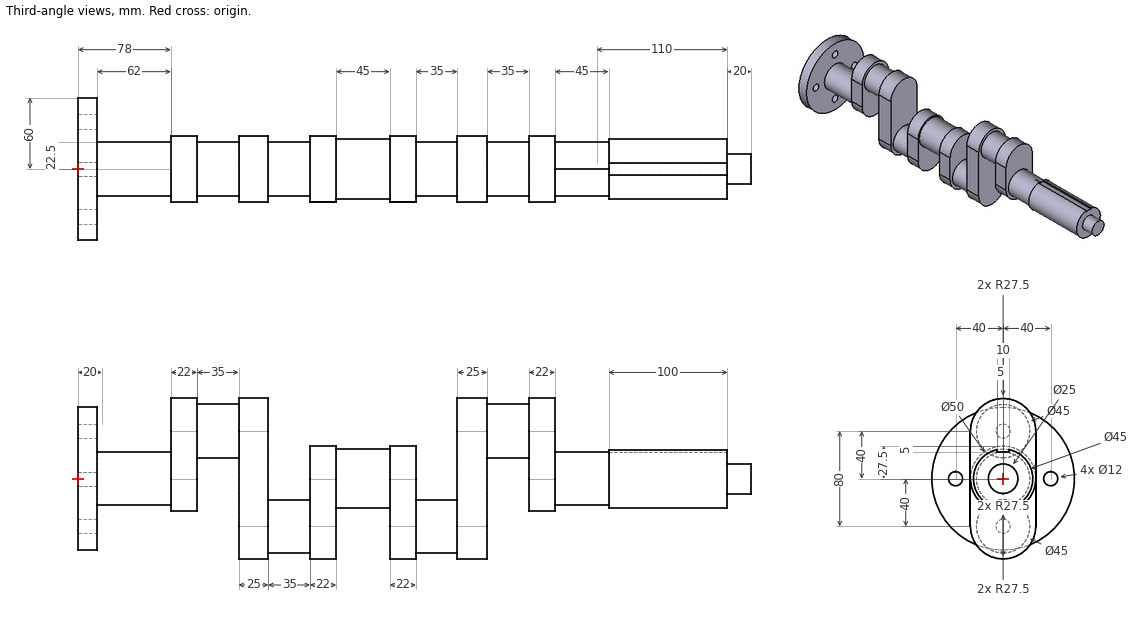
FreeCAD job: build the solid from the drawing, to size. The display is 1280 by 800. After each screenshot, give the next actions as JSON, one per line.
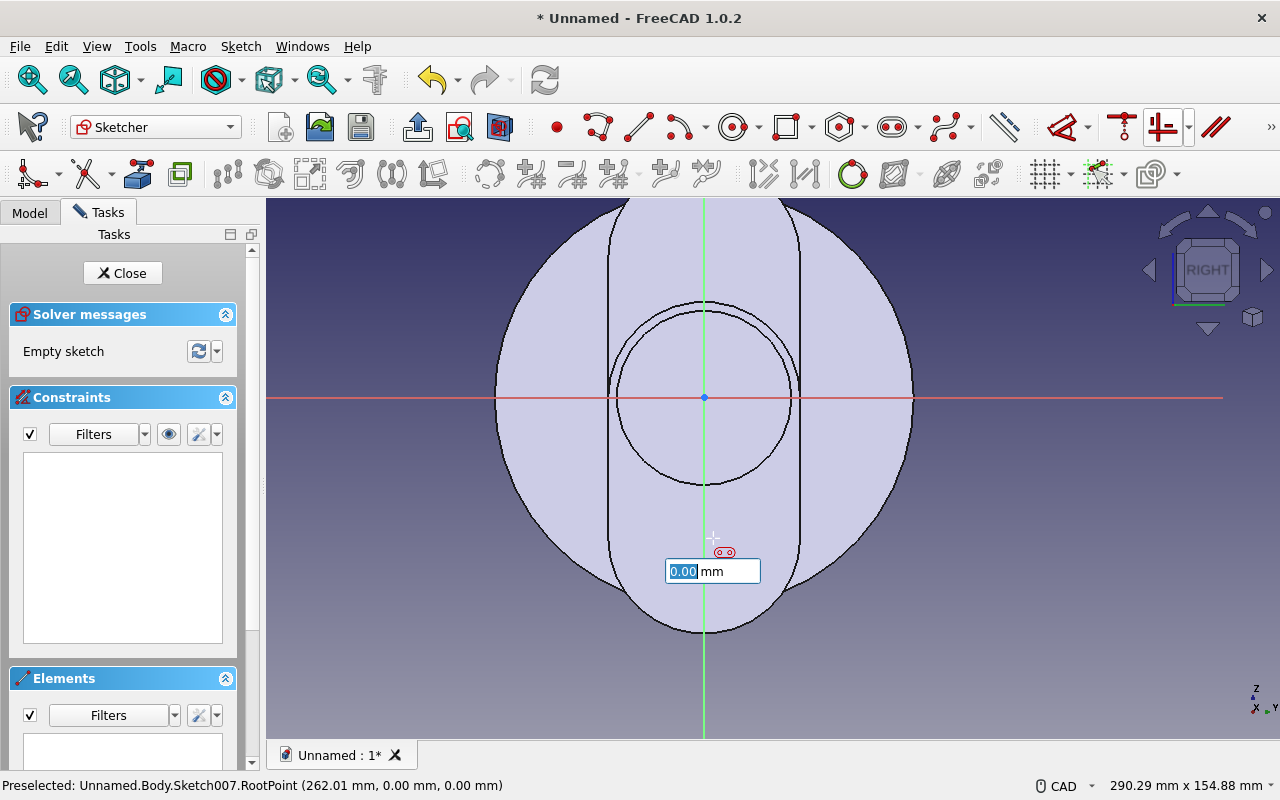
{"action": "left_click", "coordinate": [800, 468]}
{"action": "key", "text": "Escape"}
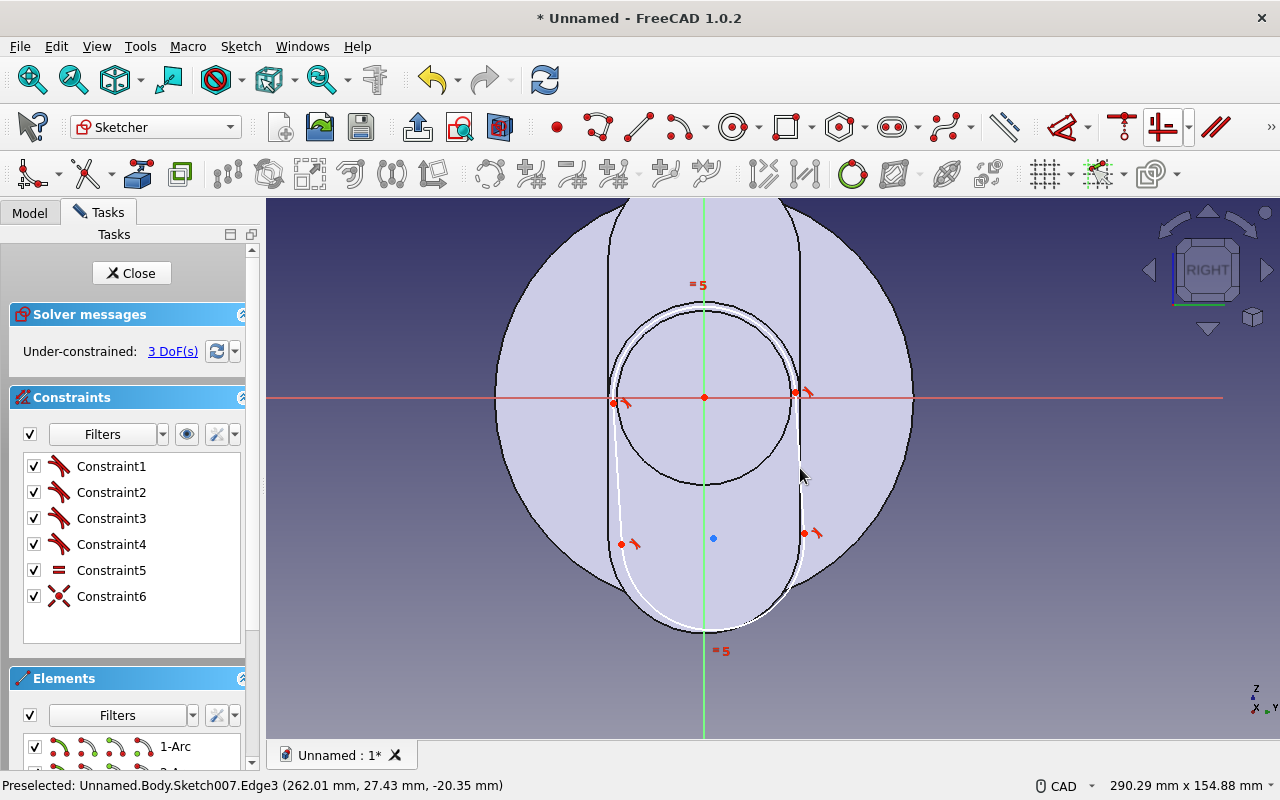
{"action": "left_click", "coordinate": [798, 435]}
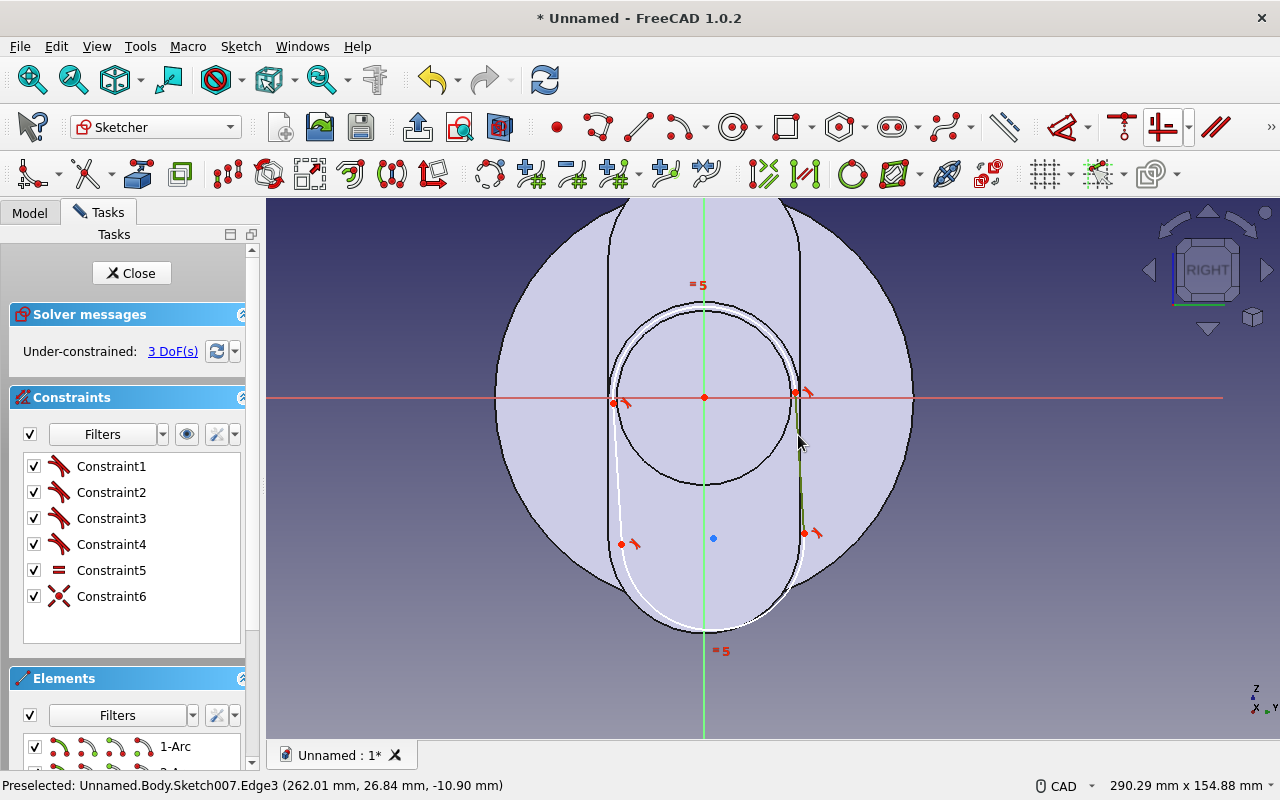
{"action": "left_click", "coordinate": [1188, 128]}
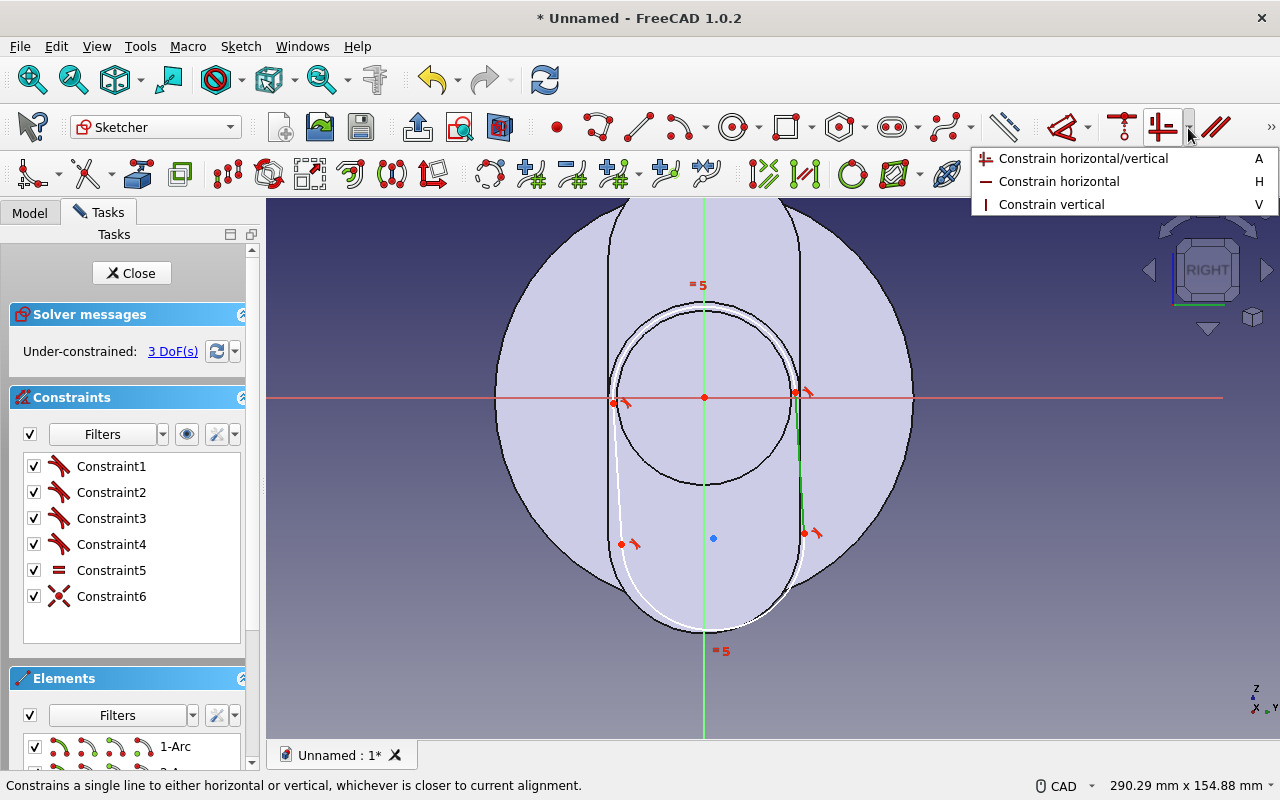
{"action": "left_click", "coordinate": [1125, 204]}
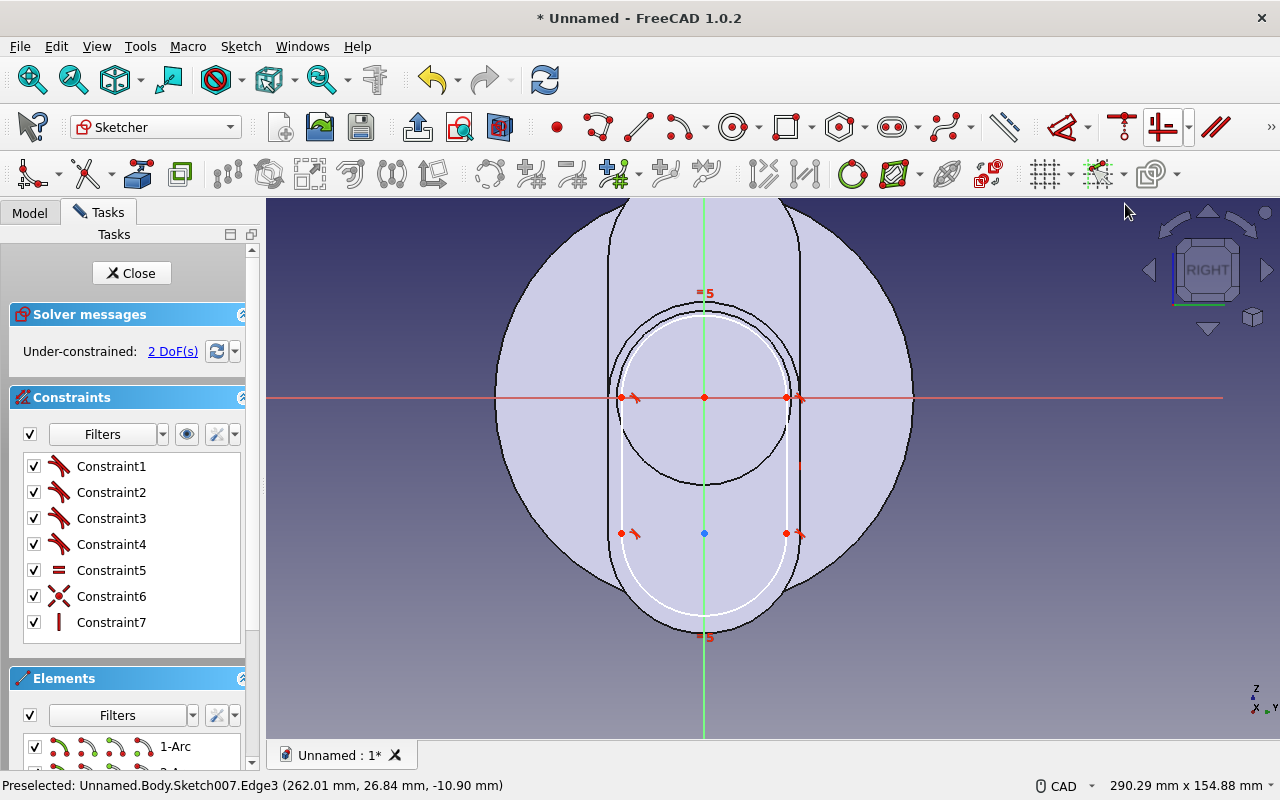
{"action": "key", "text": "d"}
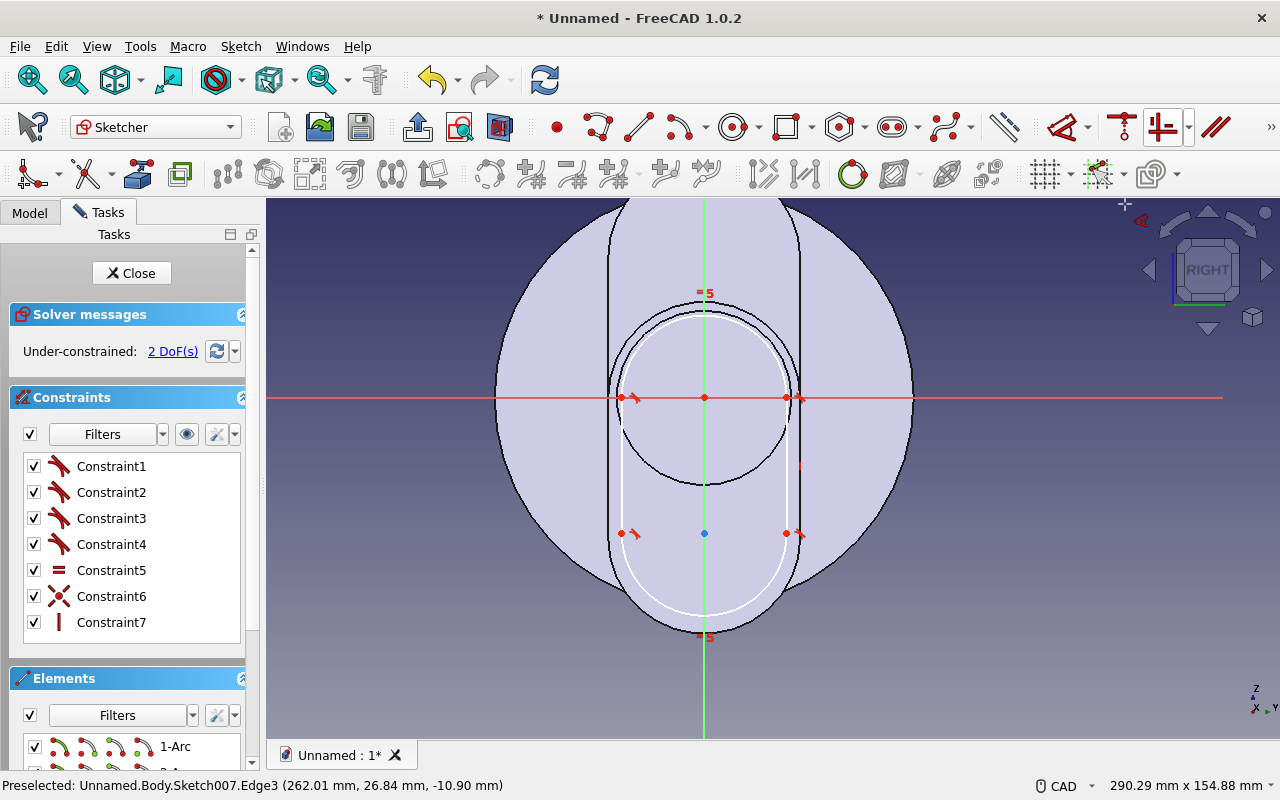
{"action": "left_click", "coordinate": [753, 331]}
{"action": "left_click", "coordinate": [772, 305]}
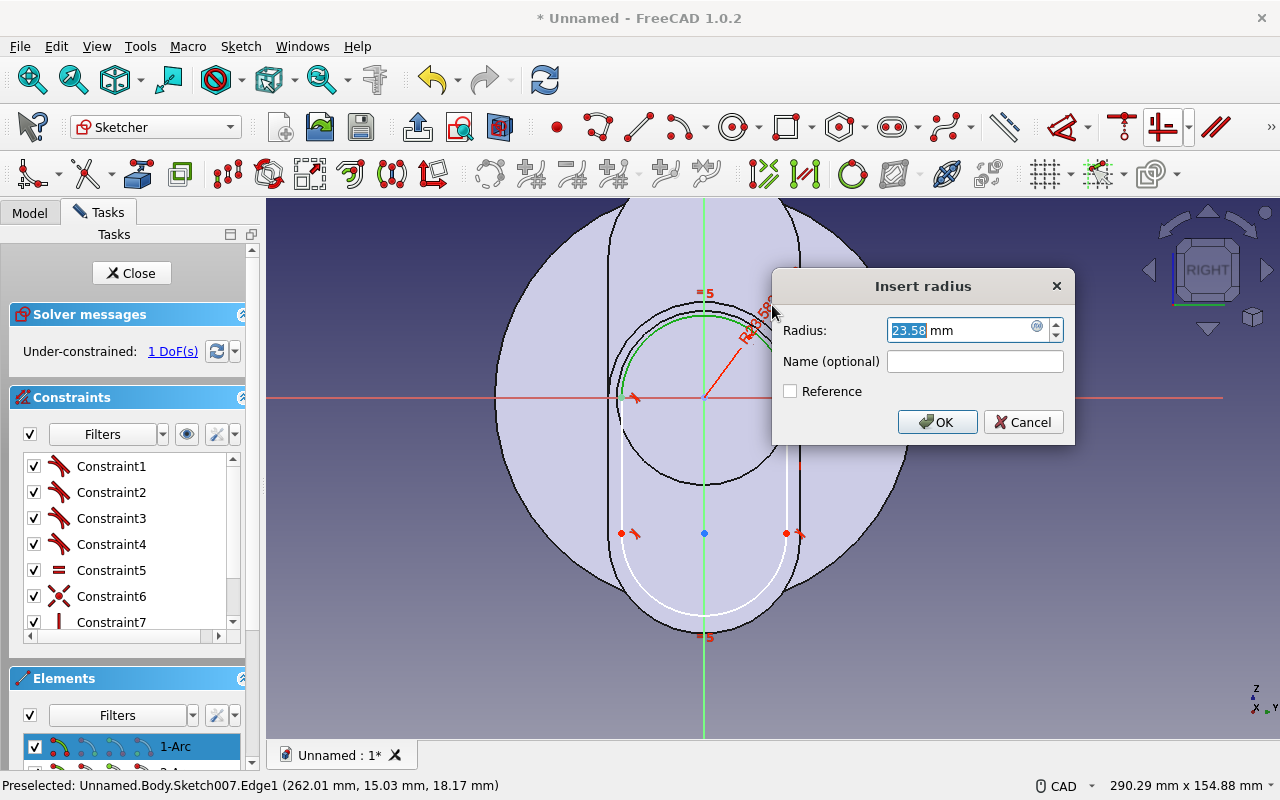
{"action": "type", "text": "27.5"}
{"action": "key", "text": "Return"}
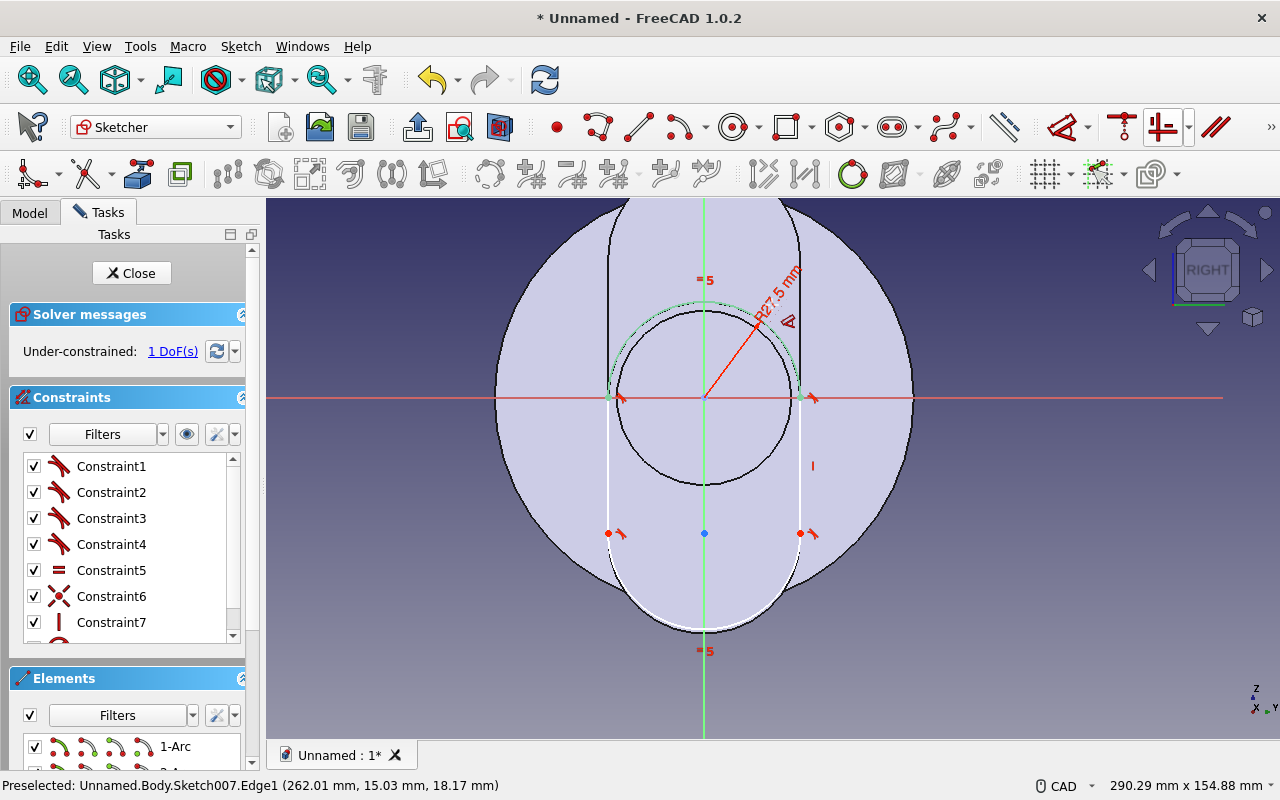
{"action": "left_click", "coordinate": [800, 439]}
{"action": "left_click", "coordinate": [834, 466]}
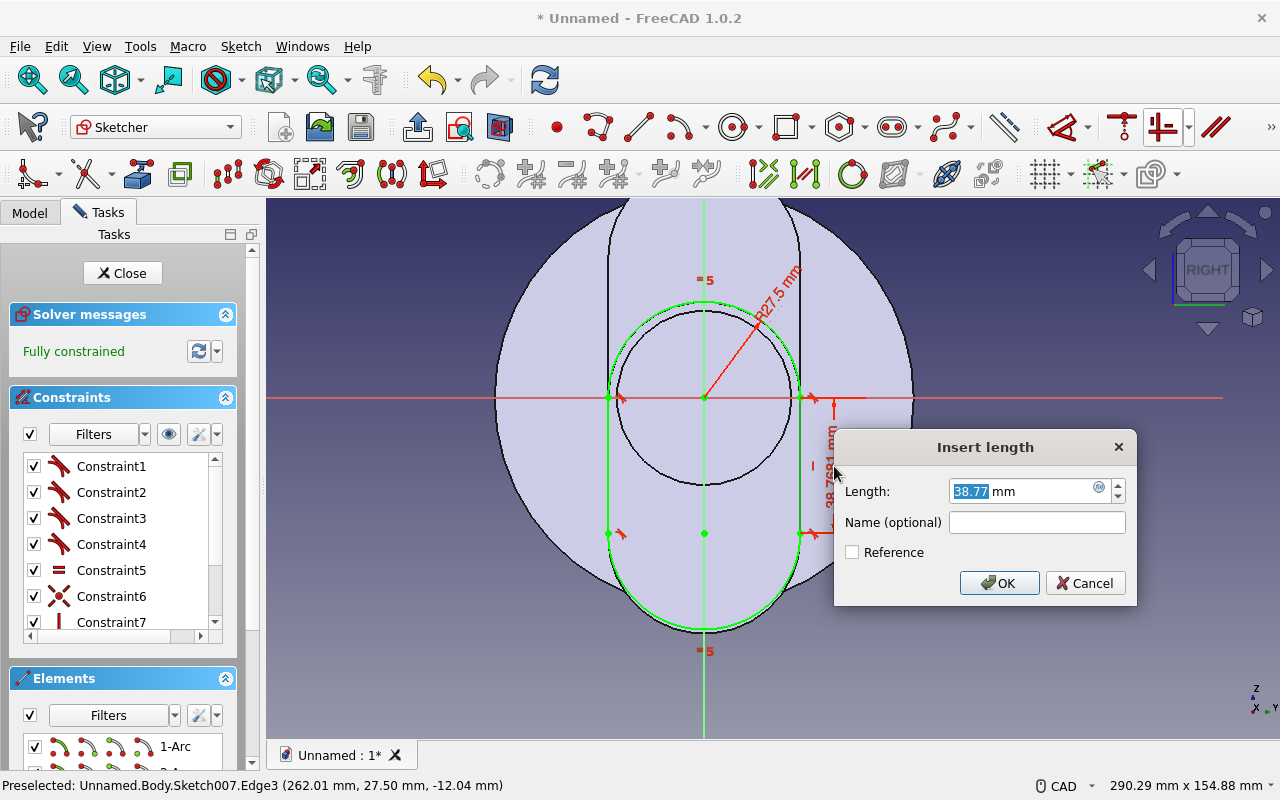
{"action": "type", "text": "40"}
{"action": "key", "text": "Return"}
{"action": "key", "text": "Escape"}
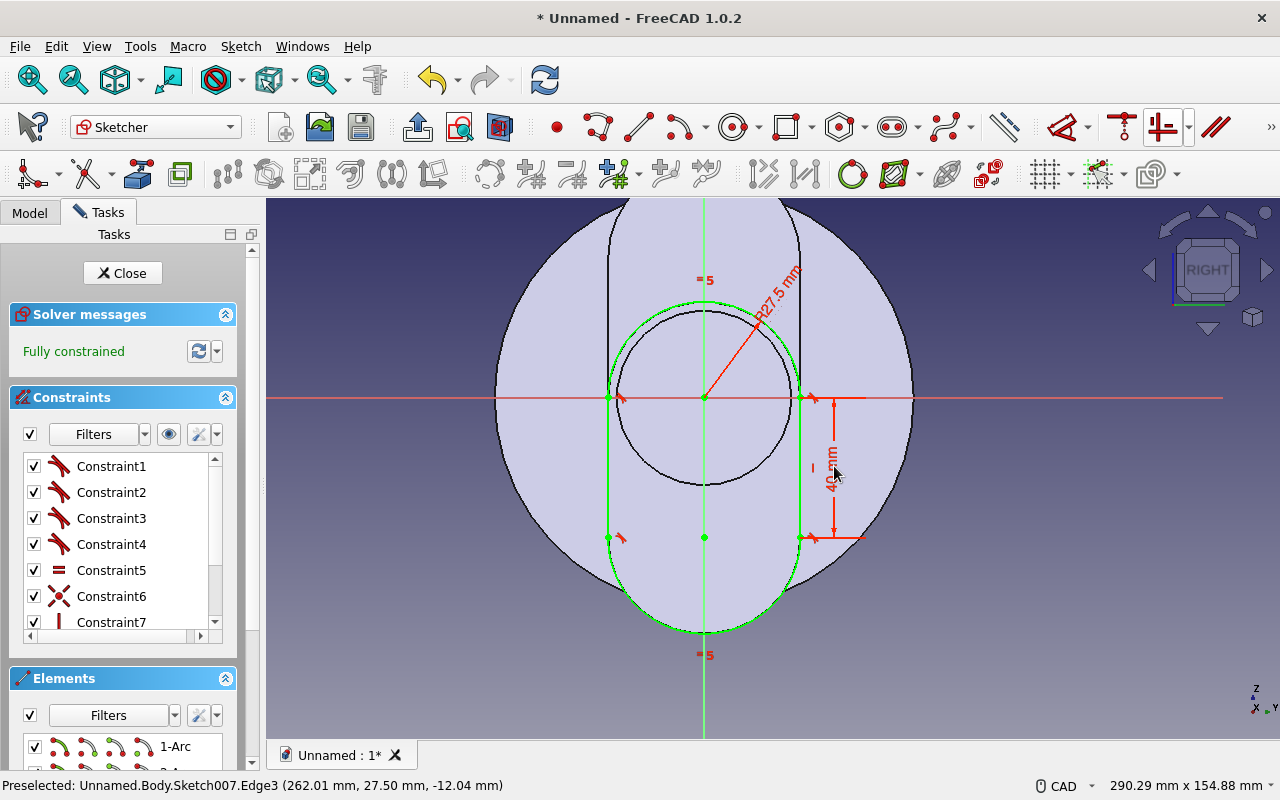
{"action": "left_click", "coordinate": [123, 273]}